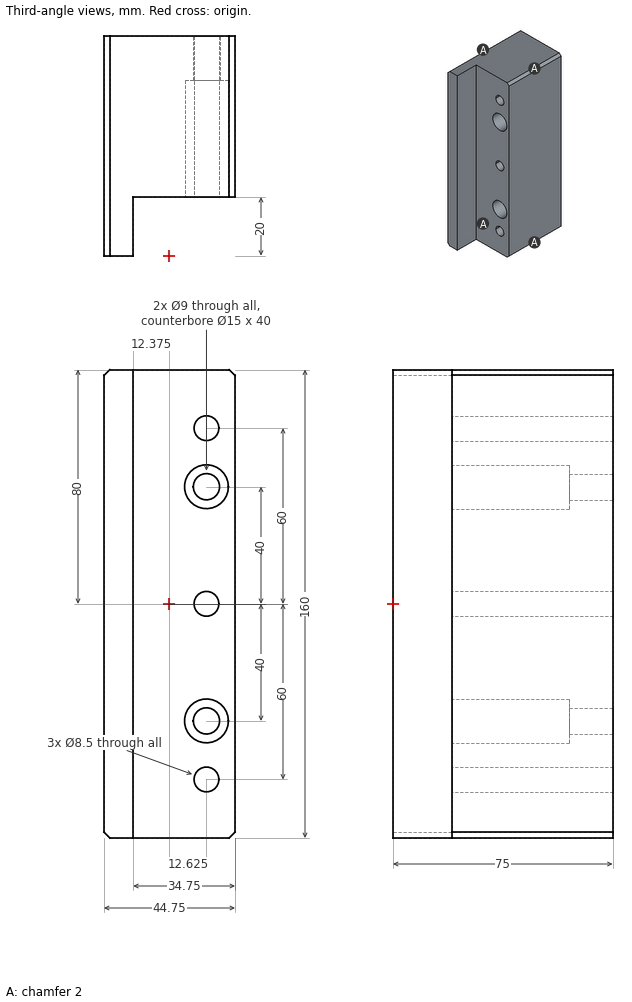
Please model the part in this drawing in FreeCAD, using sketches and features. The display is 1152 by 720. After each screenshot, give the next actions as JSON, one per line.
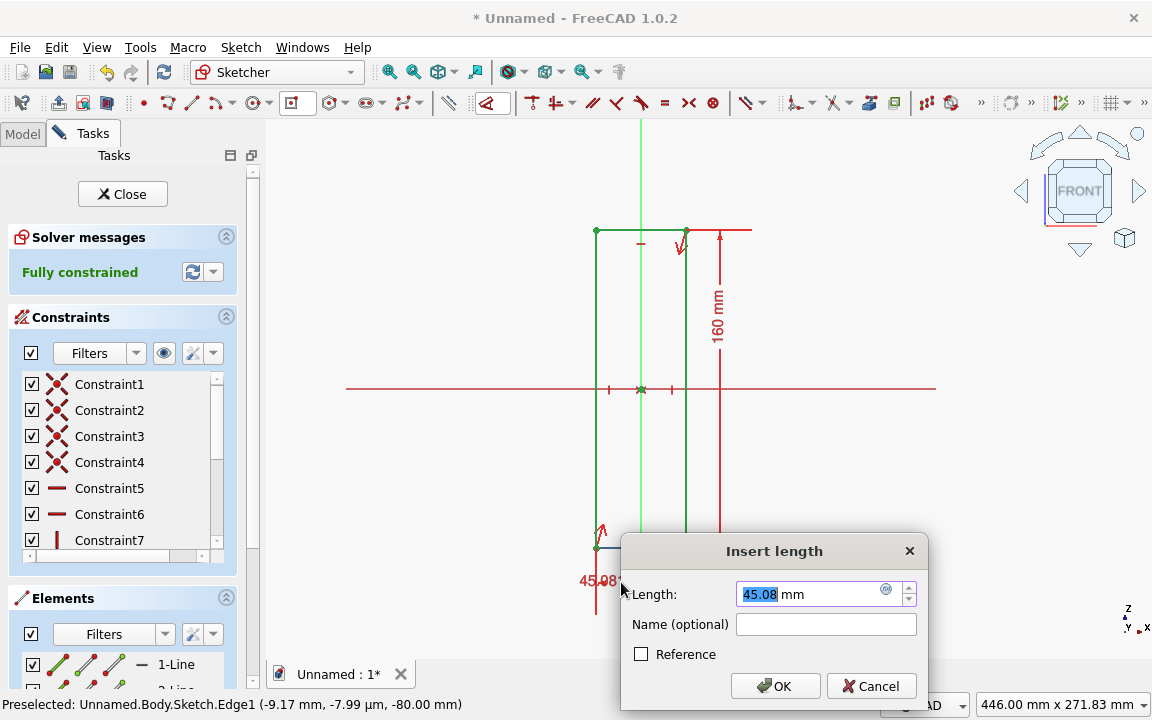
{"action": "type", "text": "44.75"}
{"action": "key", "text": "Return"}
{"action": "key", "text": "Escape"}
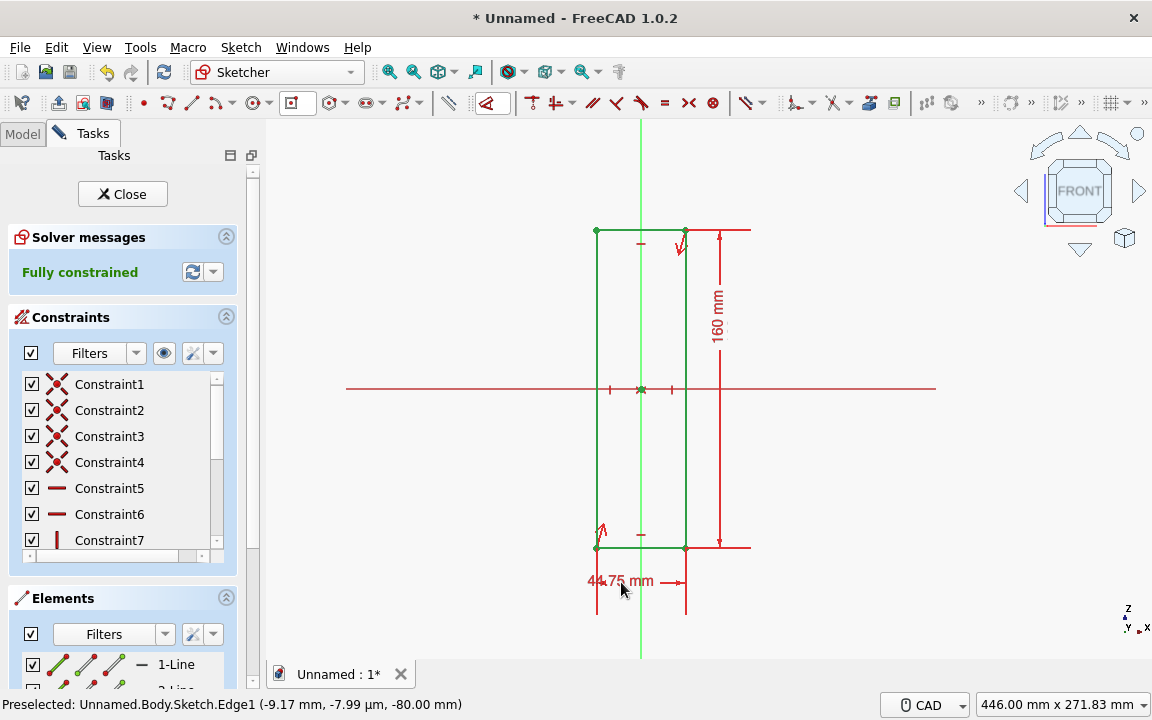
{"action": "left_click", "coordinate": [123, 194]}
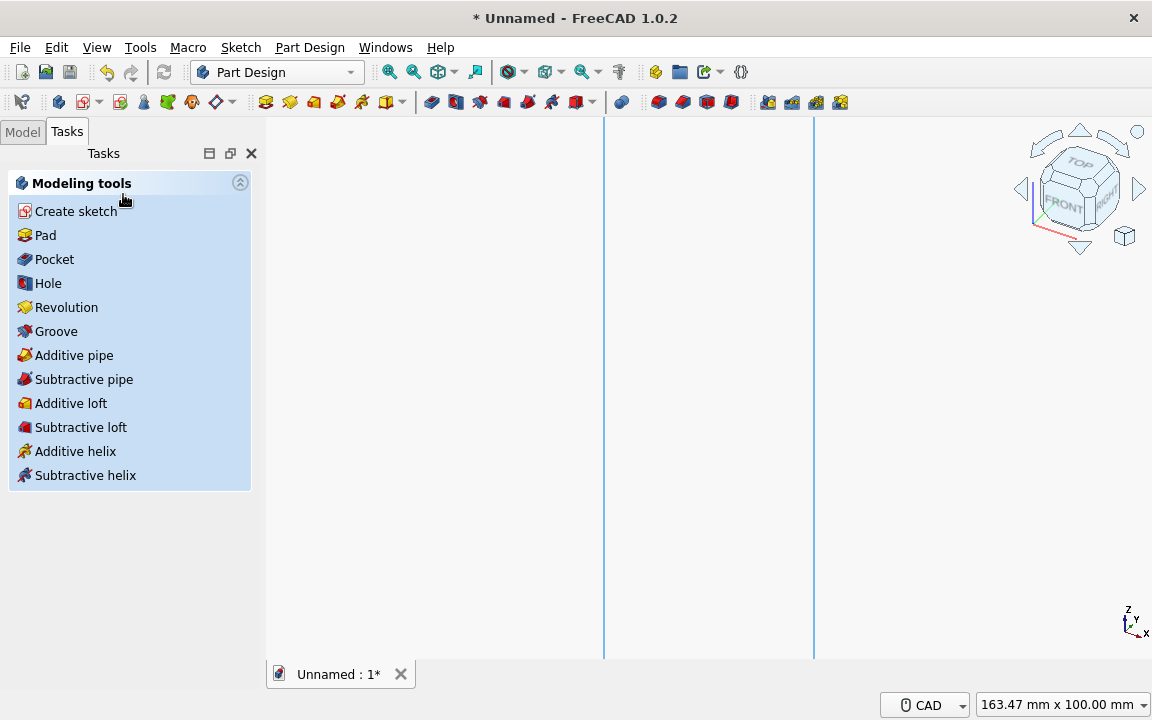
{"action": "left_click", "coordinate": [266, 102]}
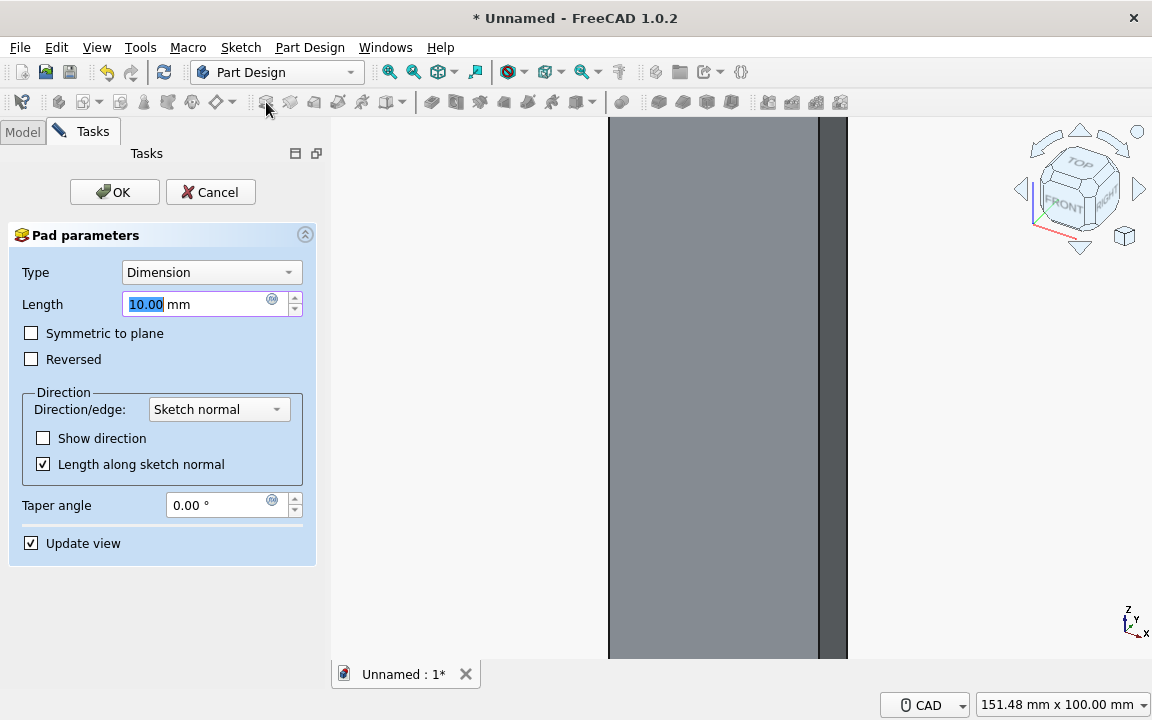
{"action": "type", "text": "75"}
{"action": "key", "text": "Tab"}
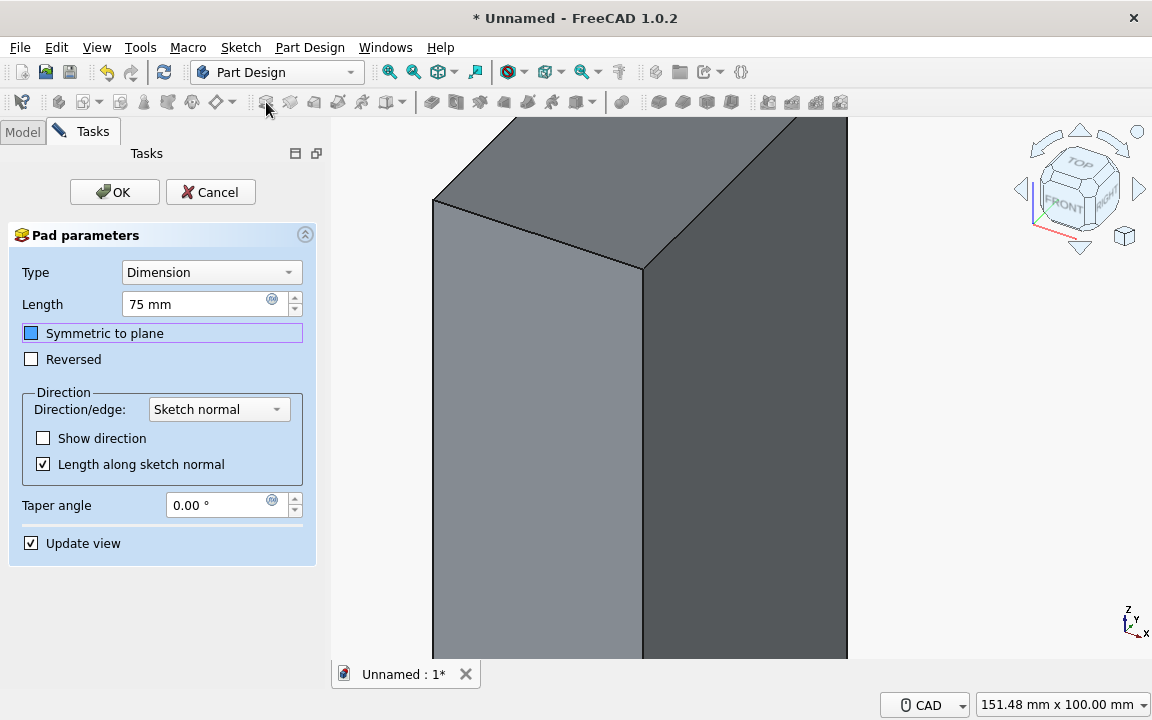
{"action": "left_click", "coordinate": [30, 359]}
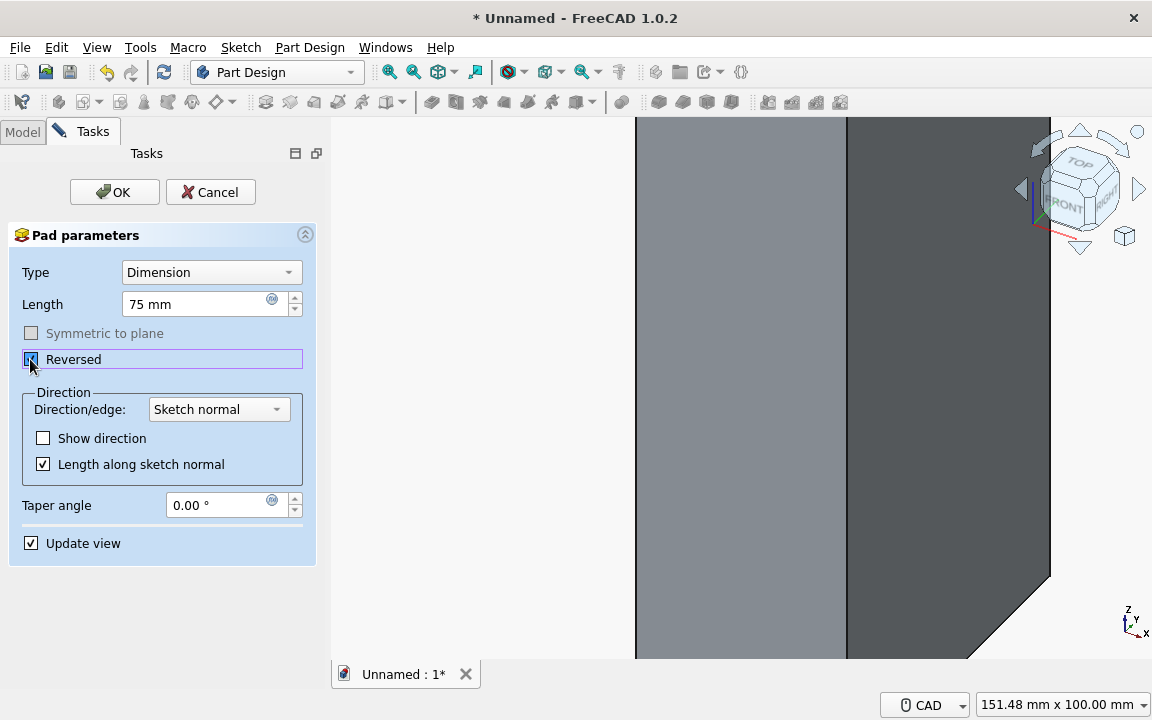
{"action": "left_click", "coordinate": [115, 192]}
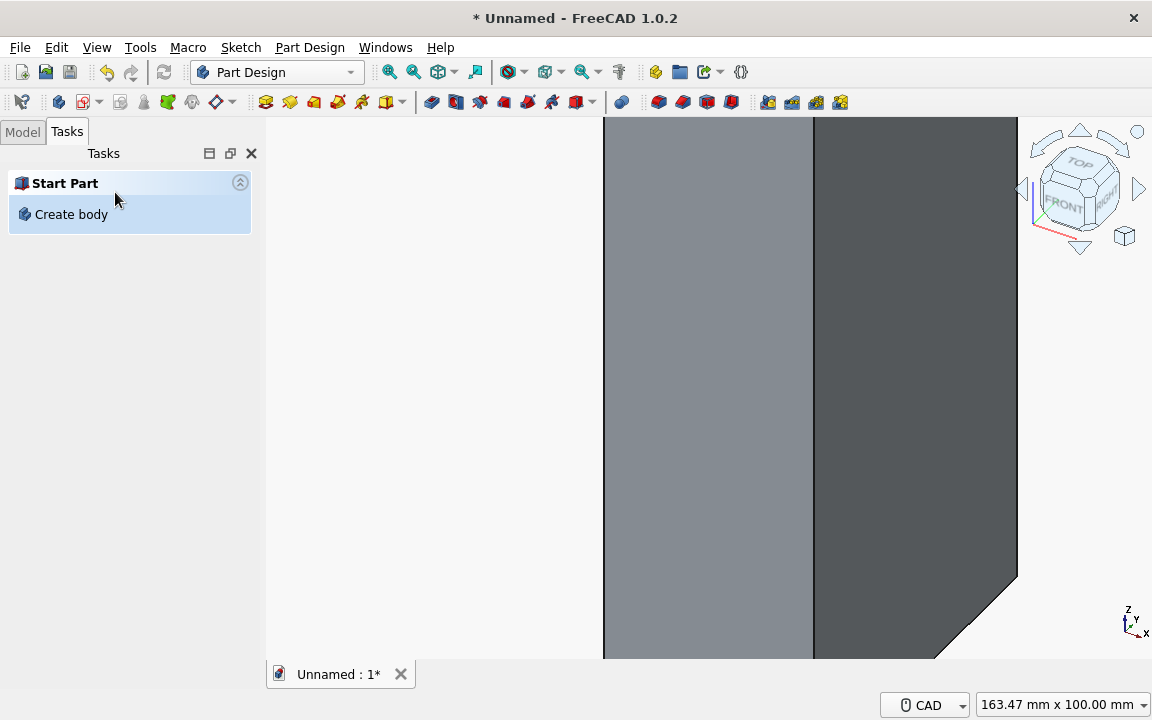
{"action": "left_click", "coordinate": [390, 72]}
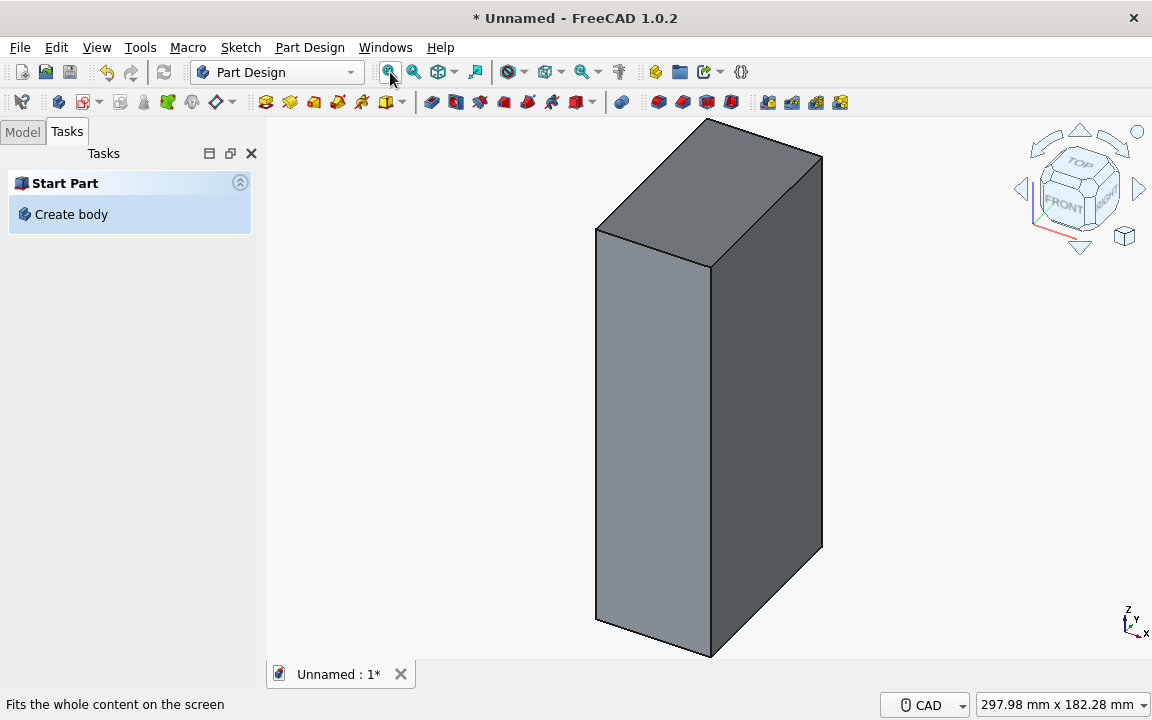
{"action": "left_click", "coordinate": [84, 102]}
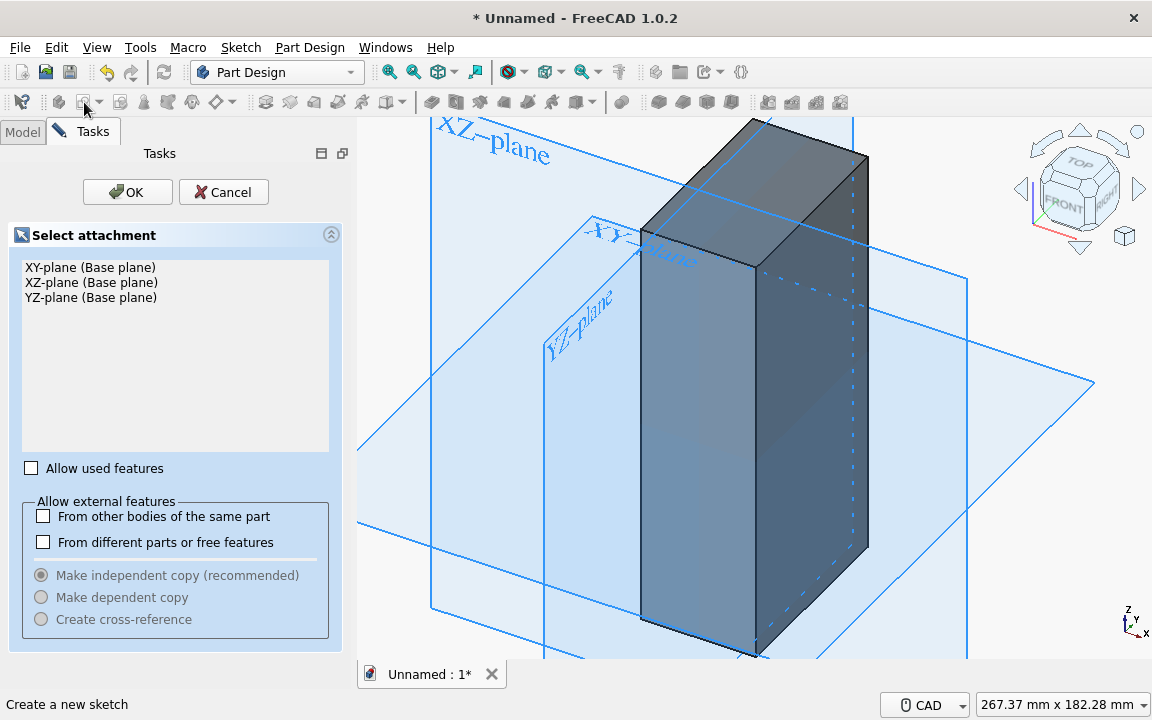
{"action": "left_click", "coordinate": [82, 282]}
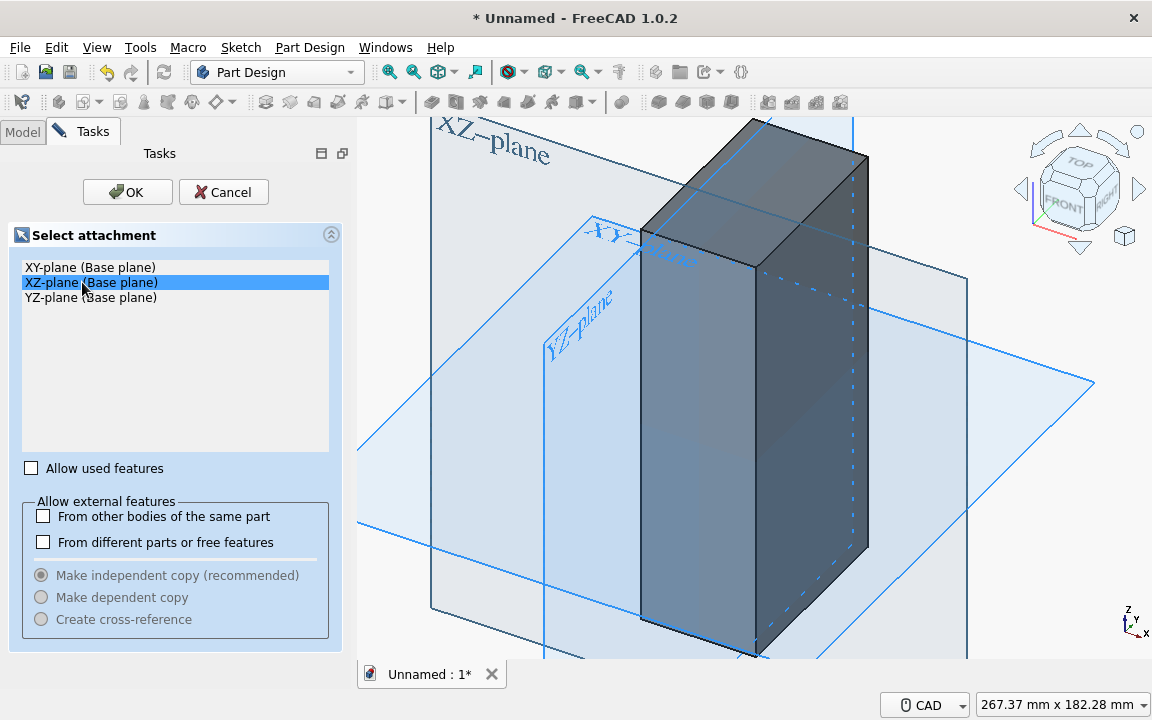
{"action": "left_click", "coordinate": [128, 192]}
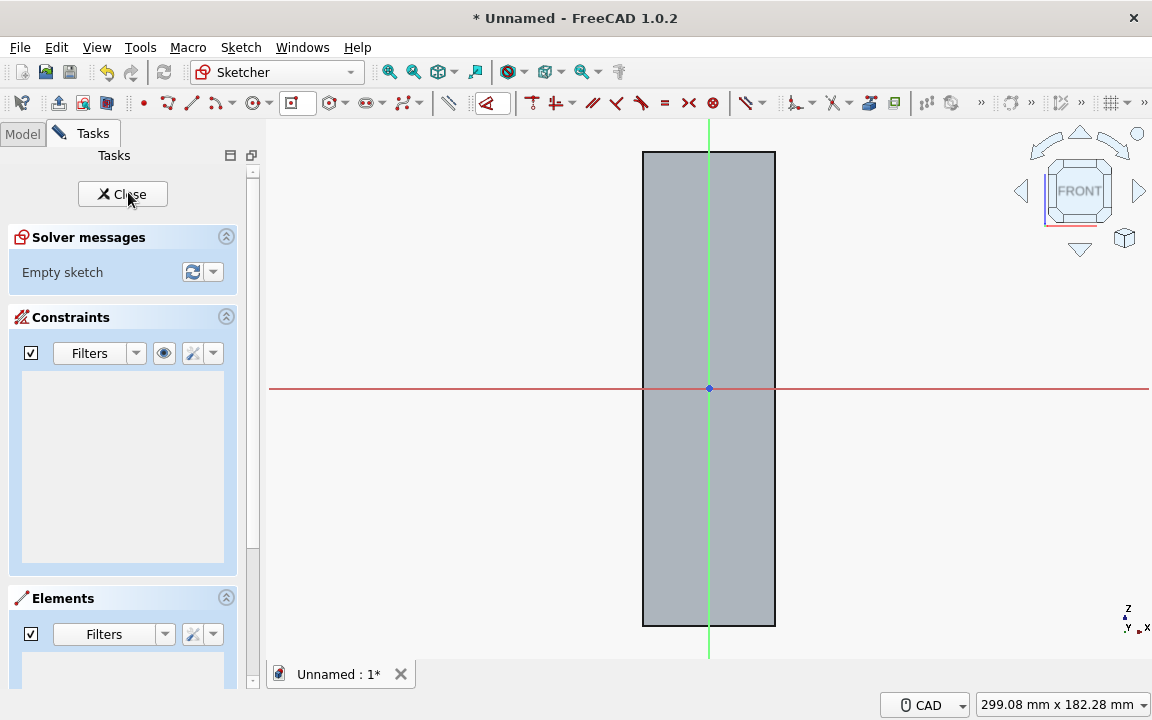
{"action": "scroll", "coordinate": [471, 389], "scroll_direction": "down", "scroll_amount": 2}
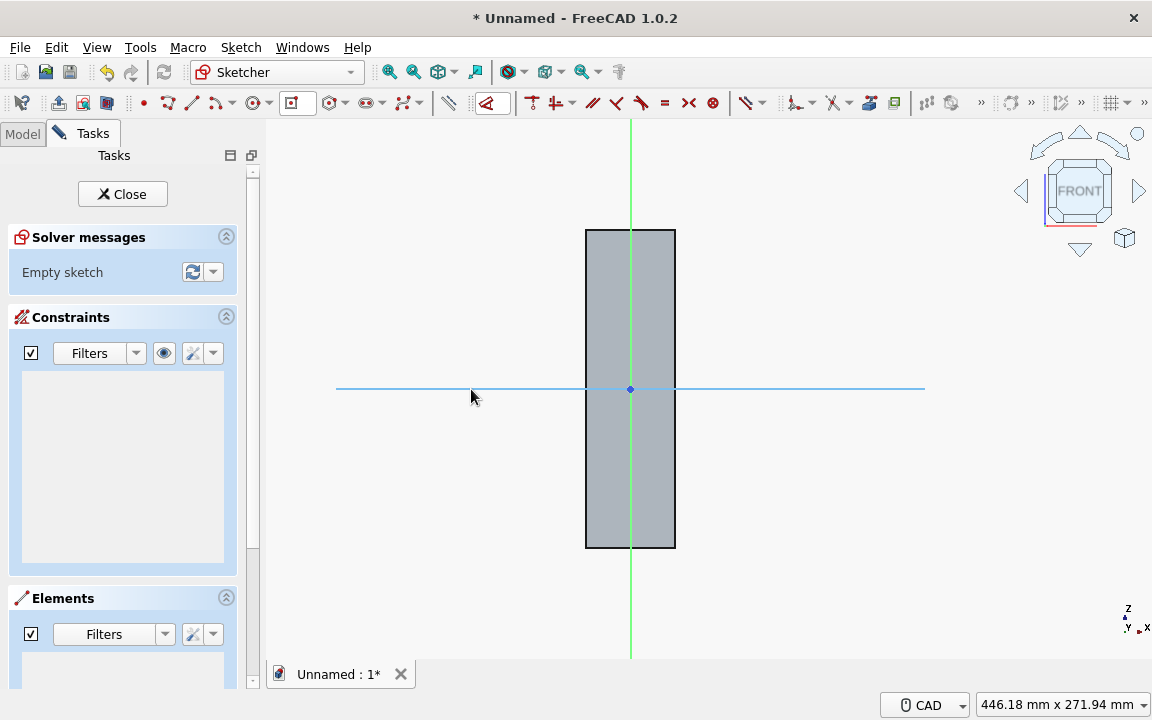
{"action": "left_click", "coordinate": [310, 104]}